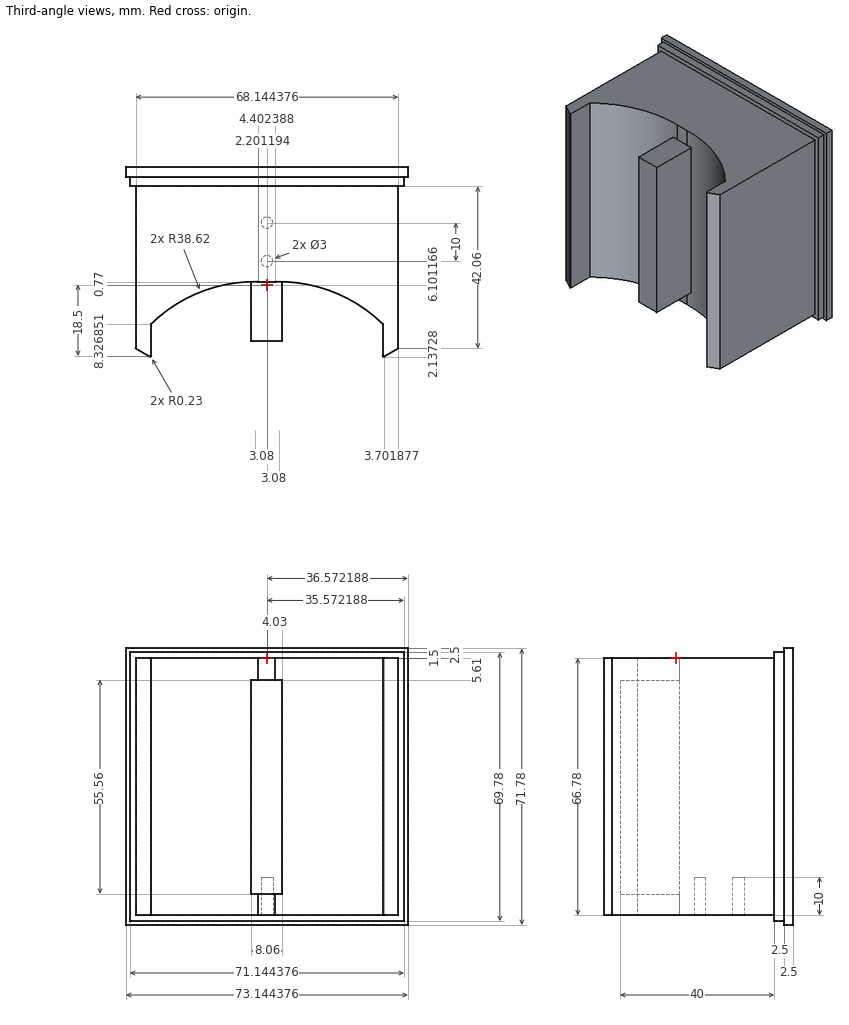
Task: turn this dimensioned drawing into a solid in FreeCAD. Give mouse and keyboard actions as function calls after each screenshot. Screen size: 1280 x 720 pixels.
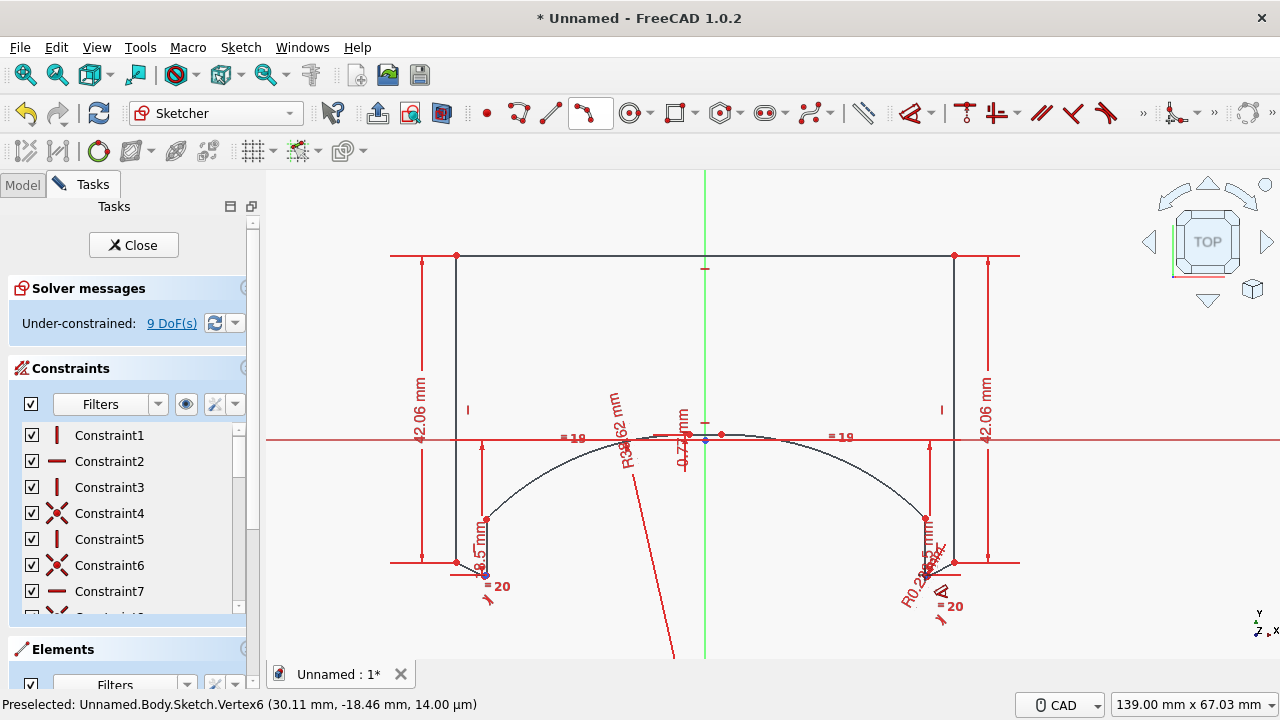
scroll(703, 270, down, 2)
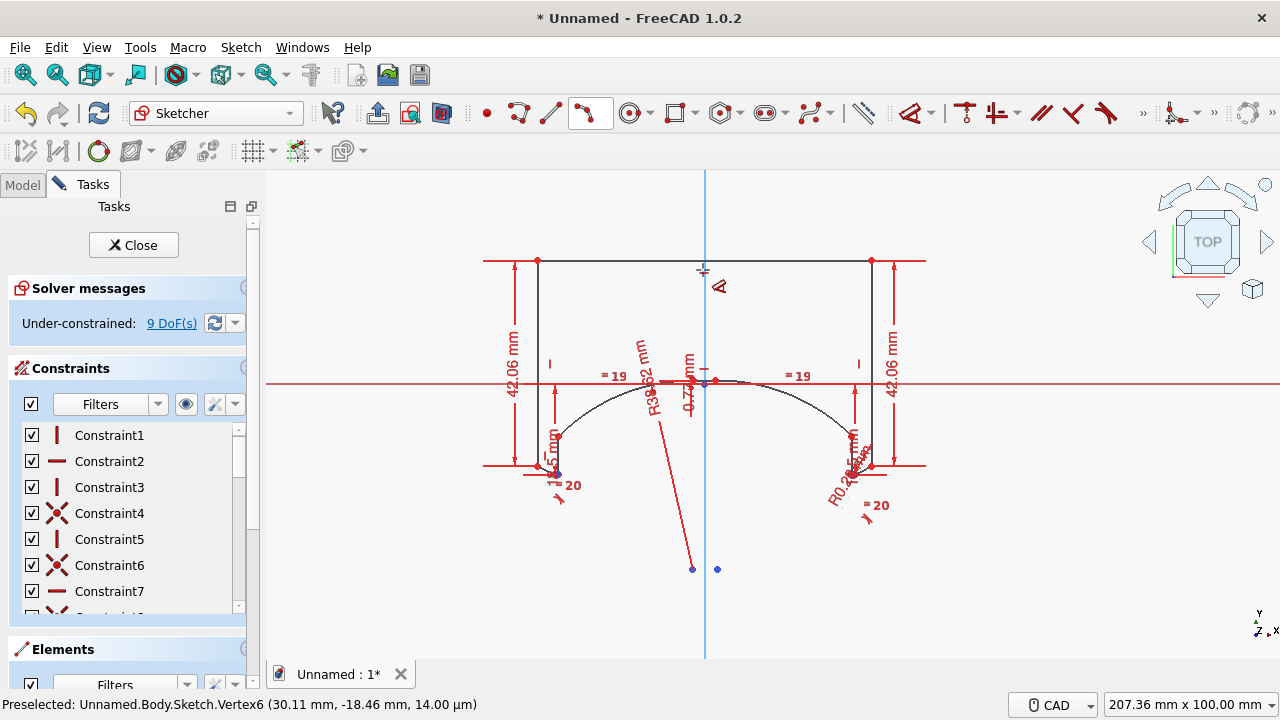
scroll(693, 569, up, 5)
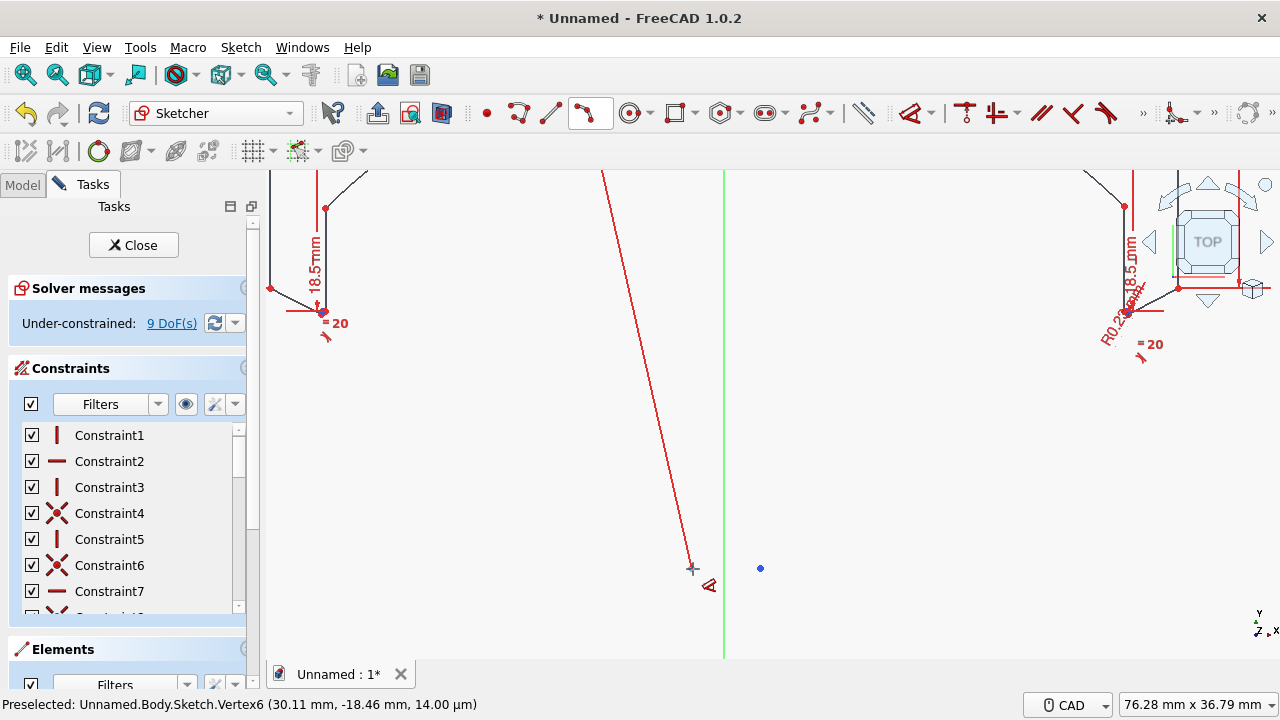
click(692, 569)
click(708, 603)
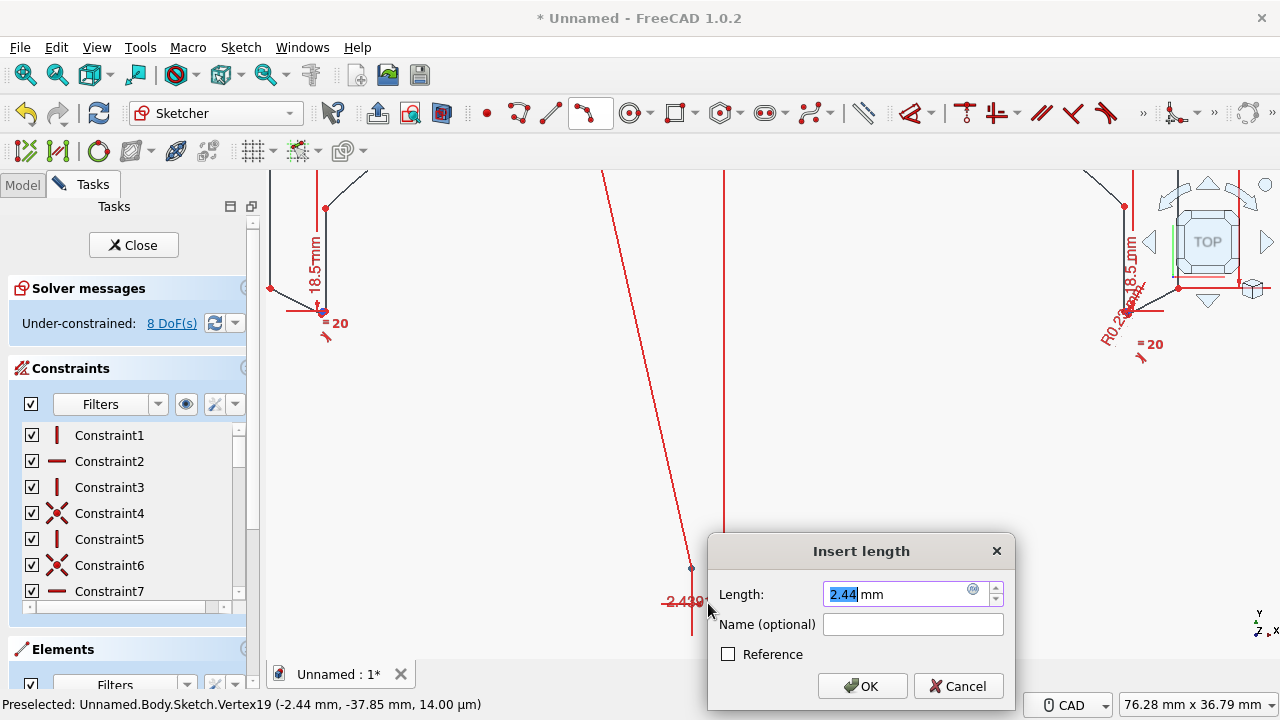
text(3.08)
key(Return)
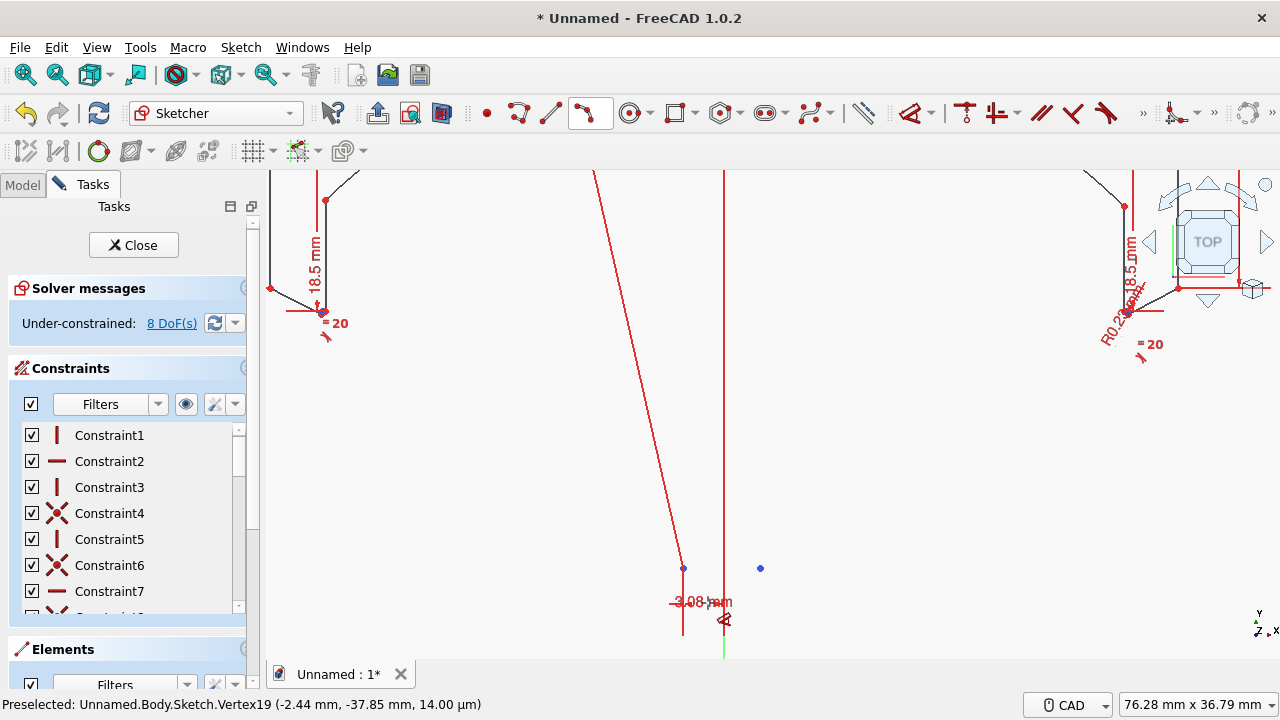
click(760, 569)
click(742, 627)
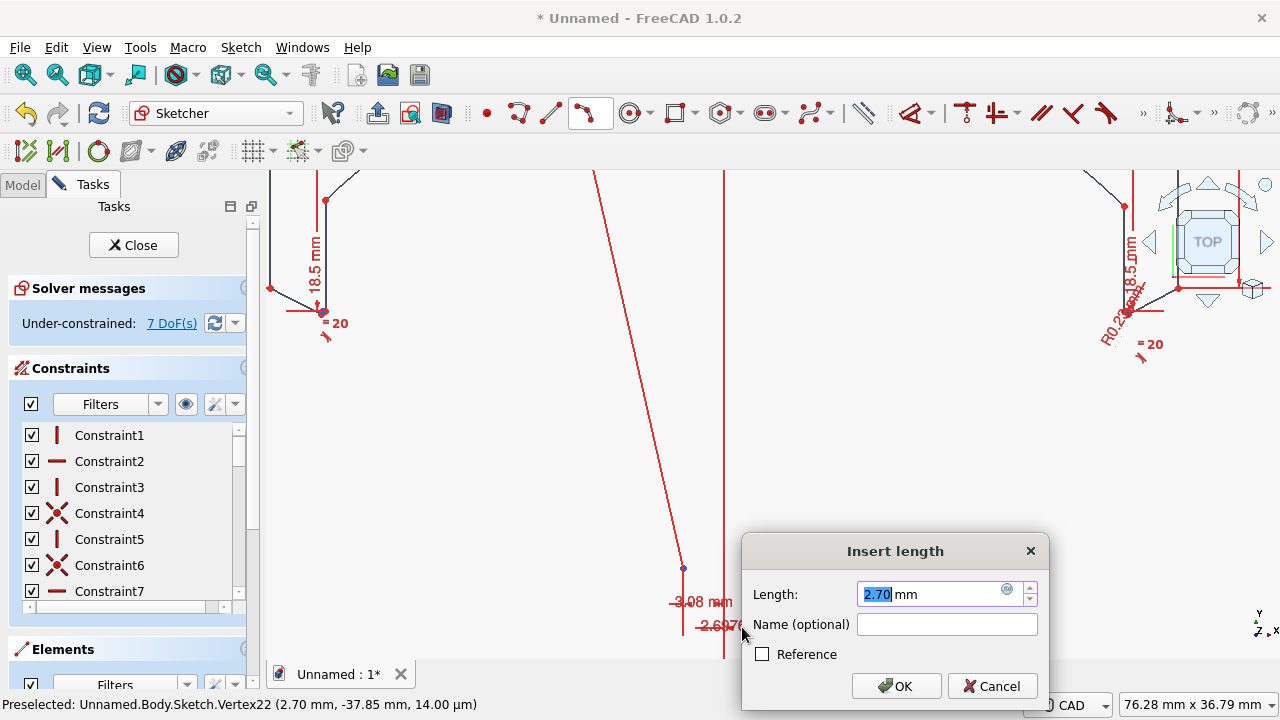
text(3.08)
key(Return)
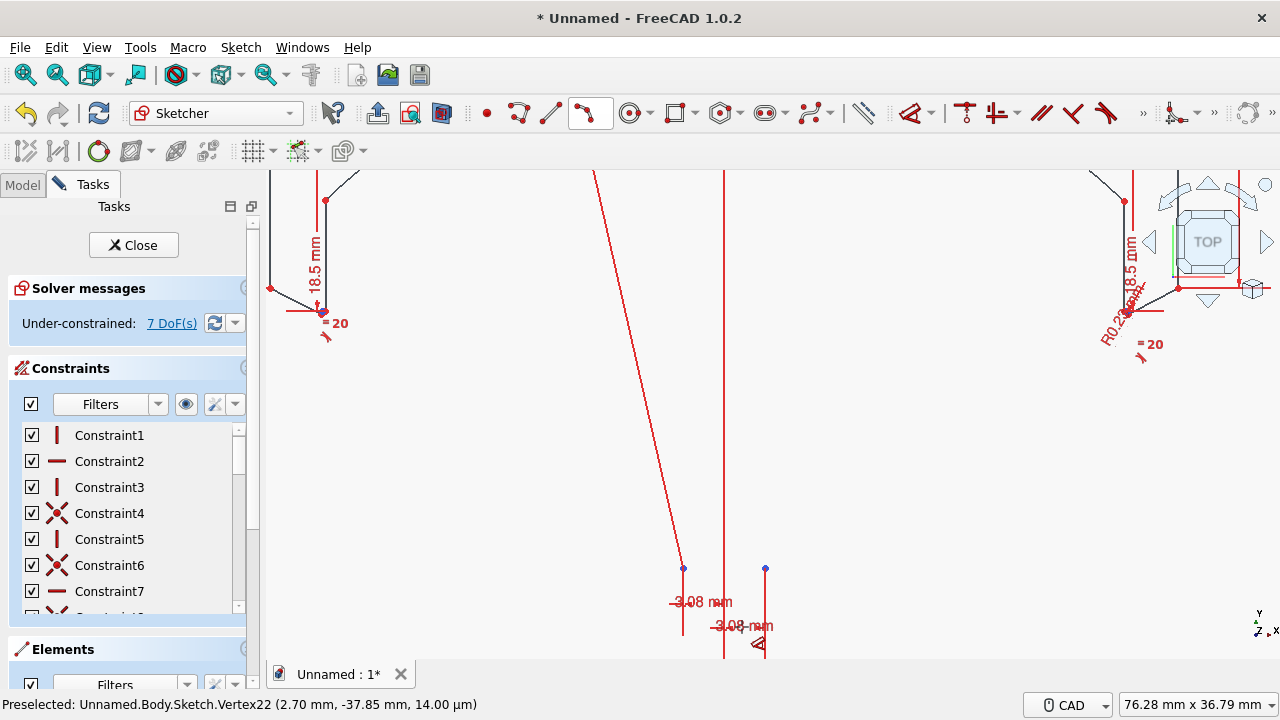
click(326, 278)
click(360, 230)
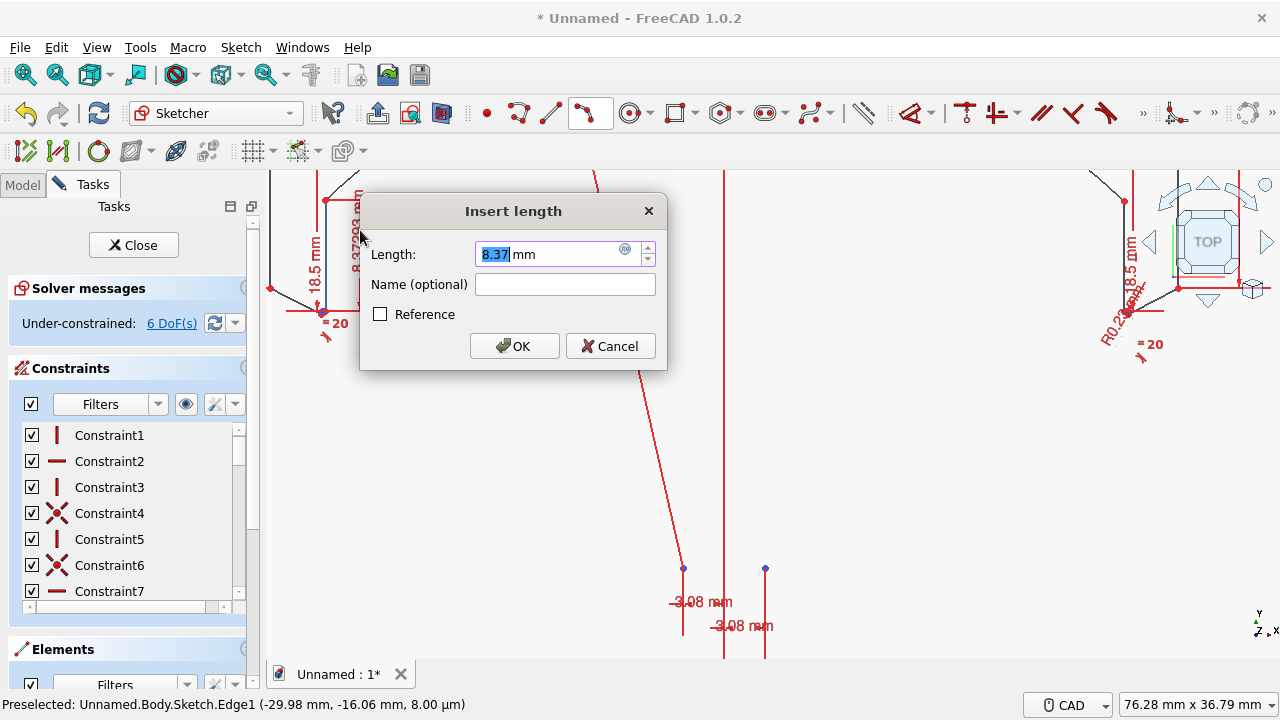
text(8.326851)
key(Return)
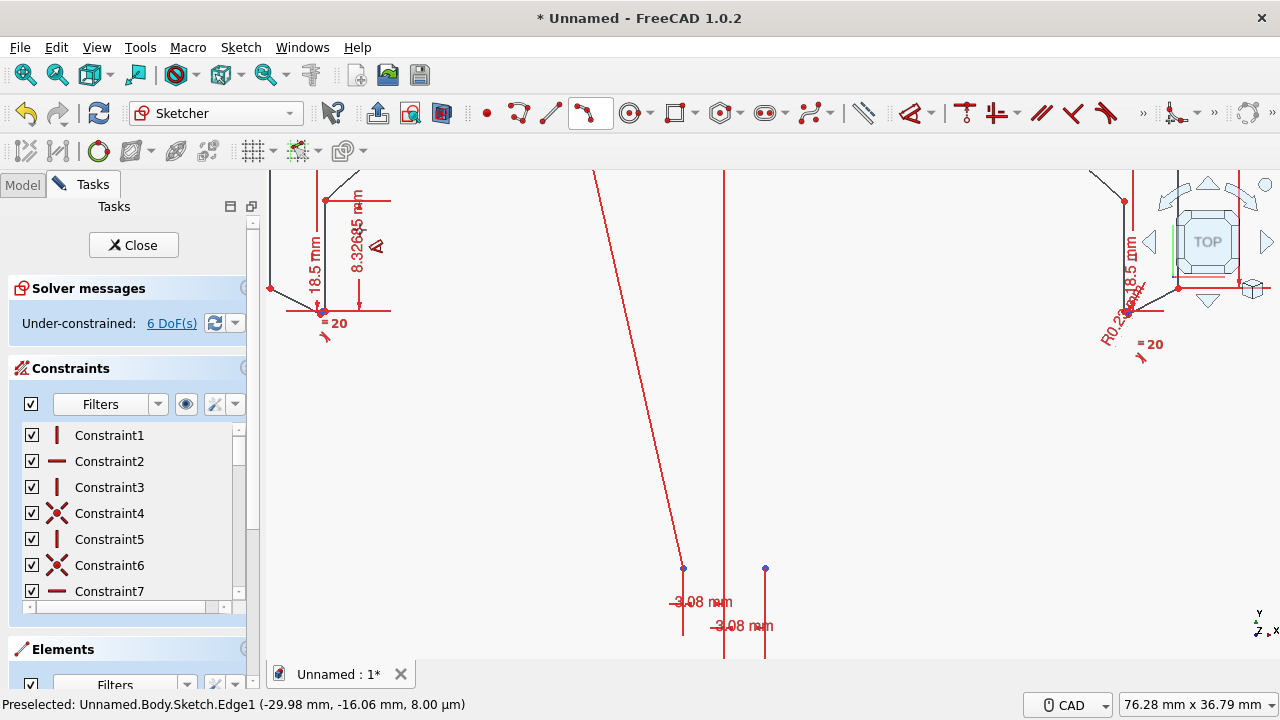
scroll(688, 631, down, 4)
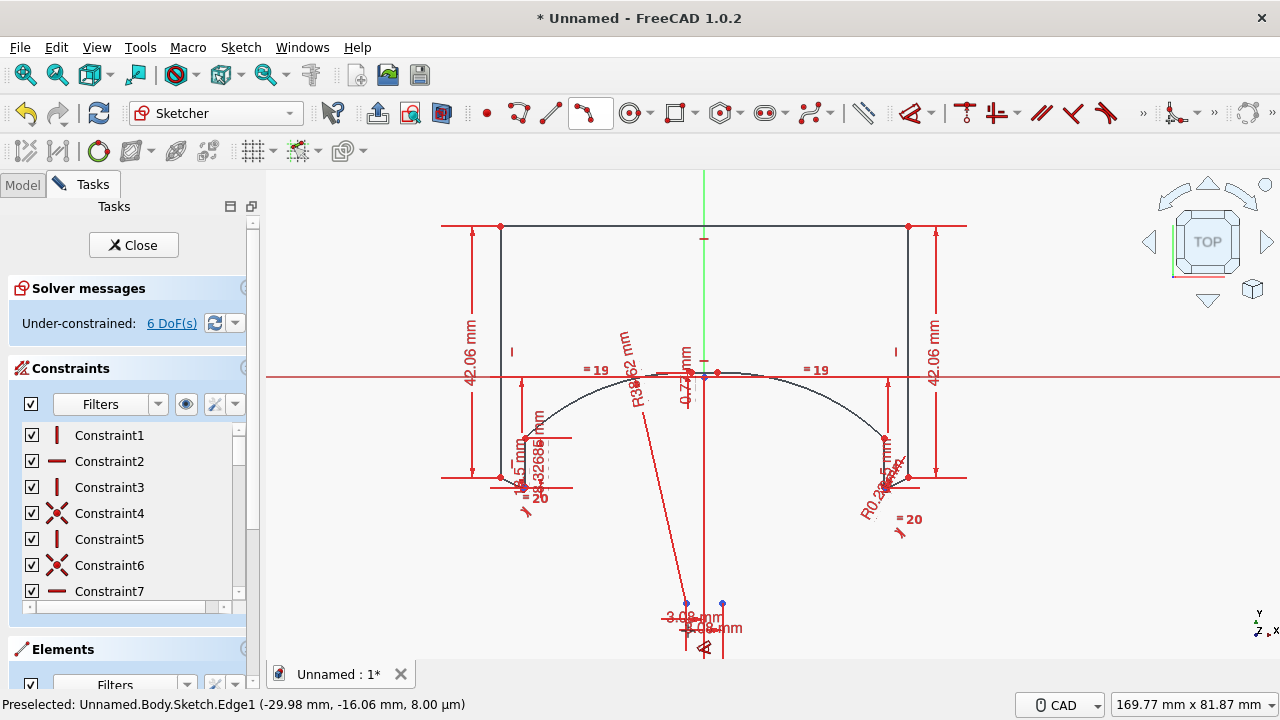
scroll(699, 373, up, 6)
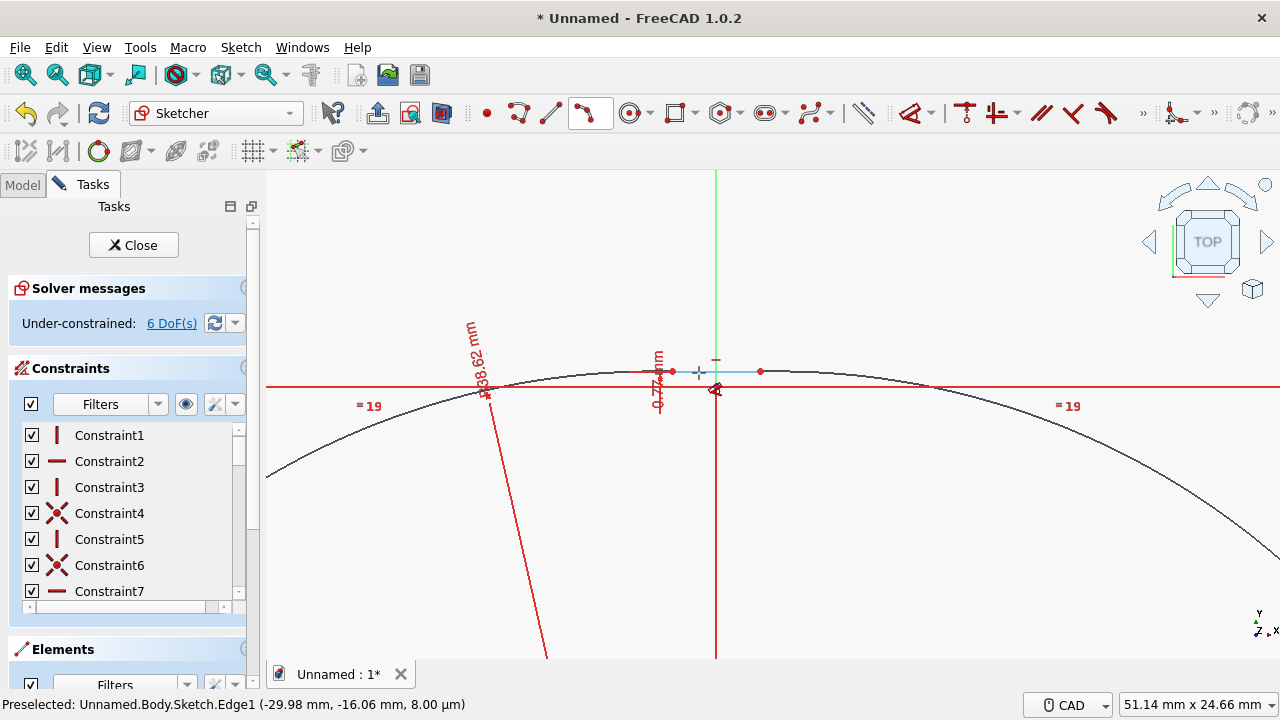
click(699, 372)
click(696, 406)